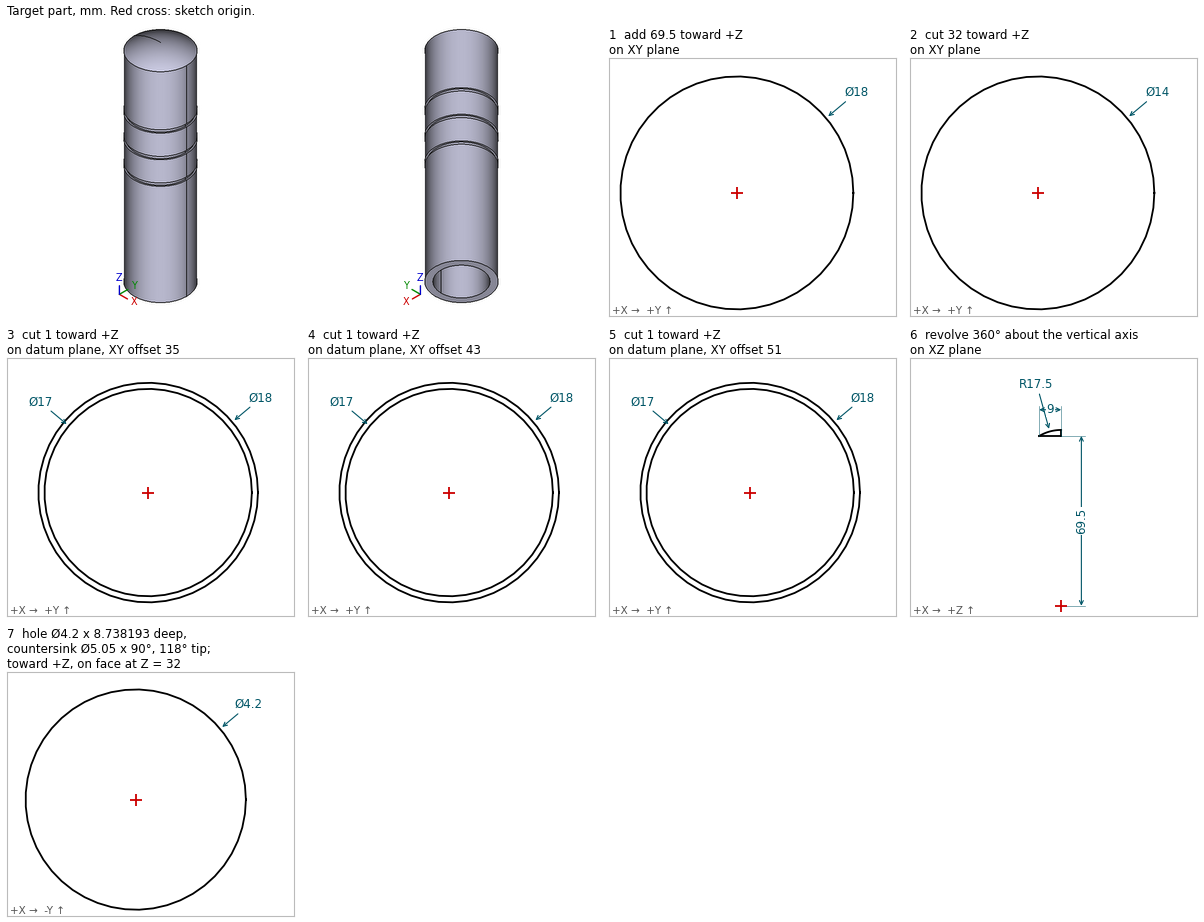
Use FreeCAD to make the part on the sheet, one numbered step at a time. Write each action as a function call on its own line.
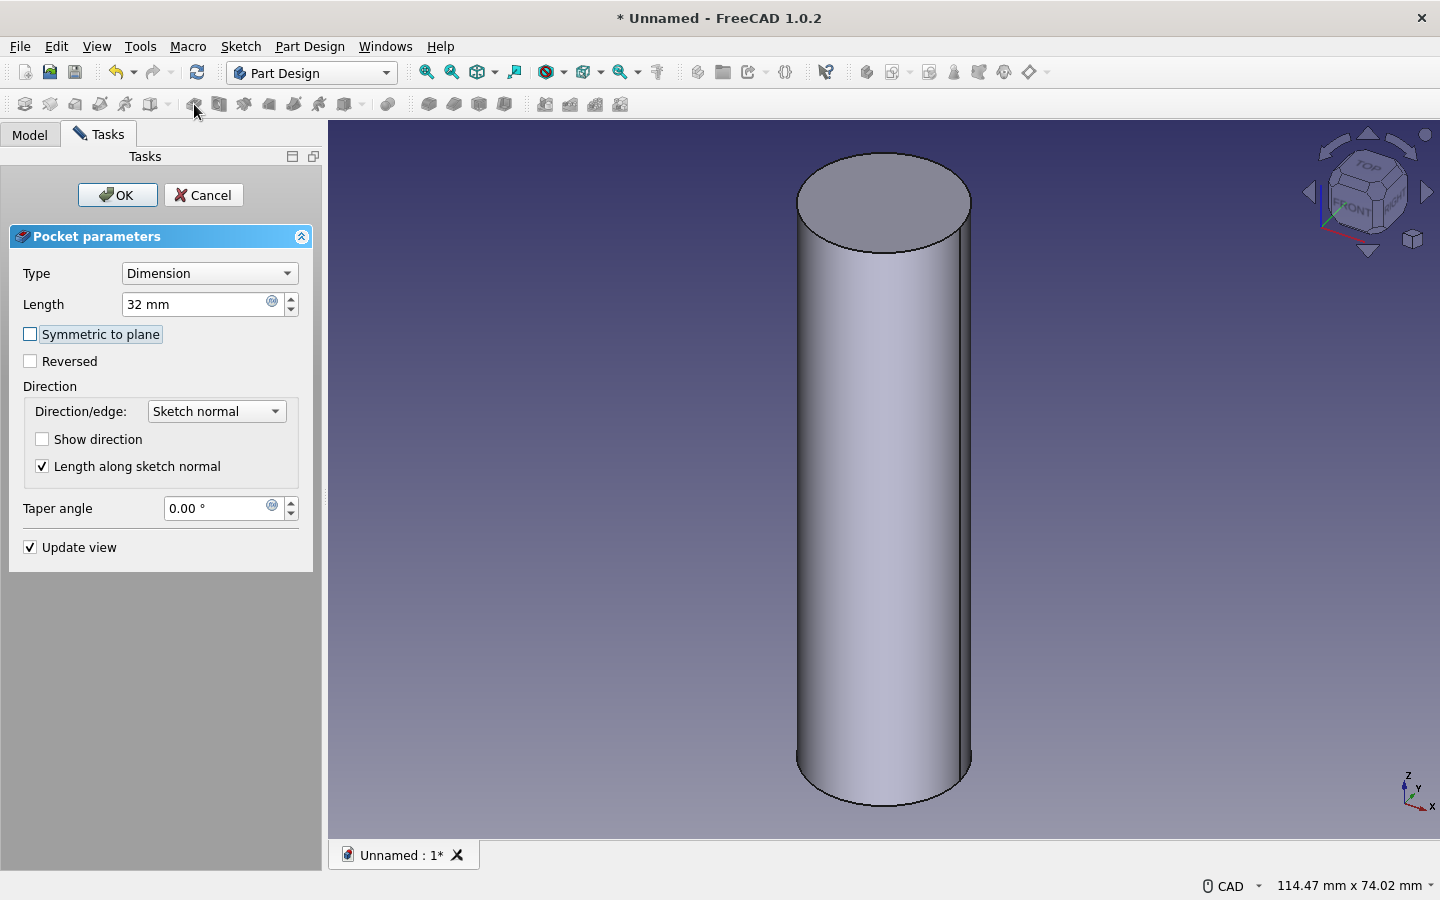
click(31, 361)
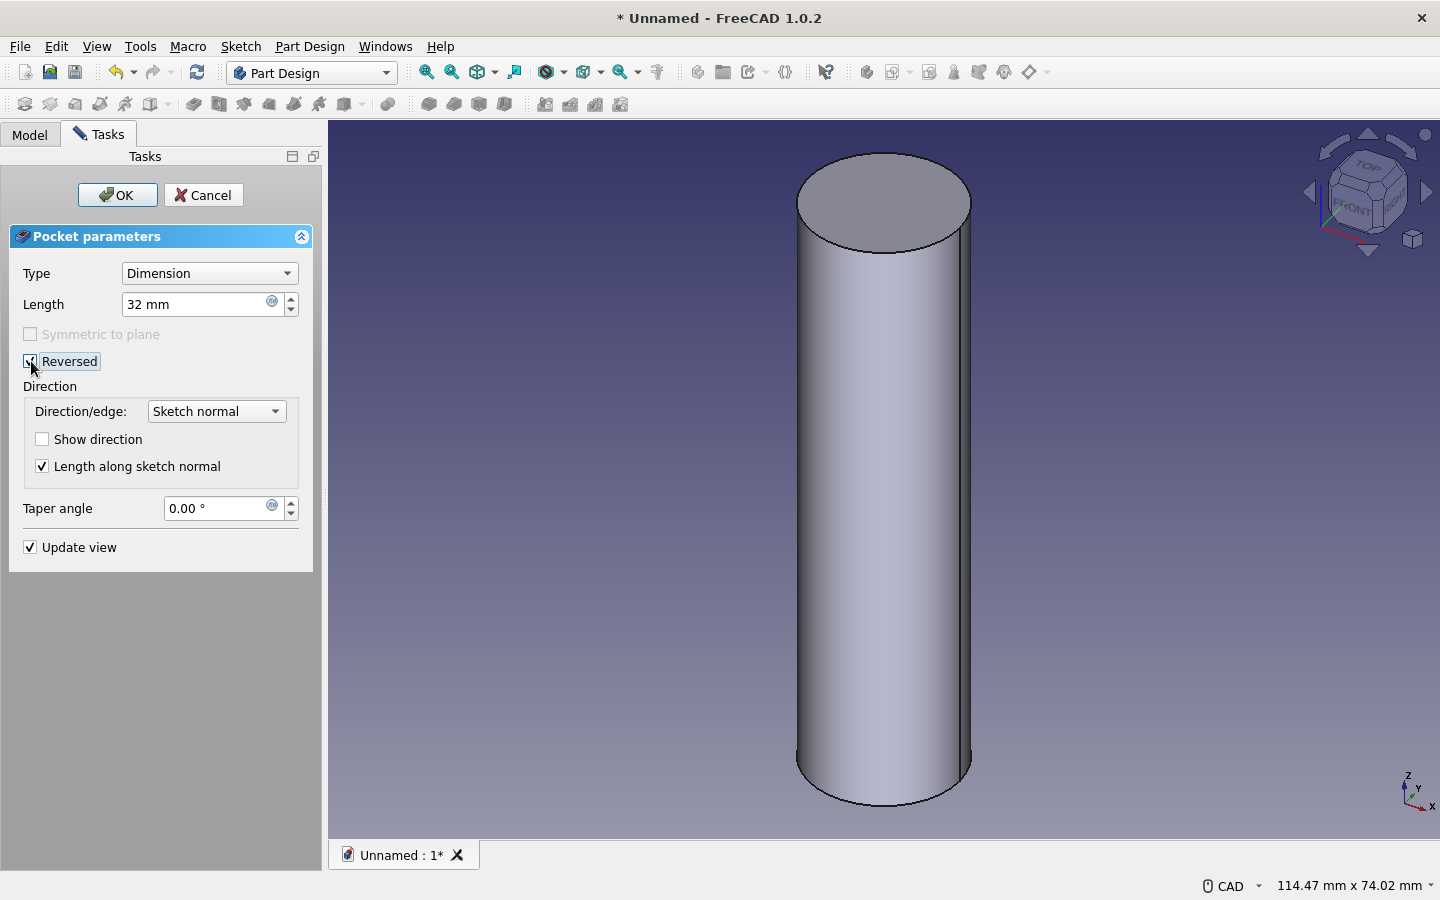
click(118, 195)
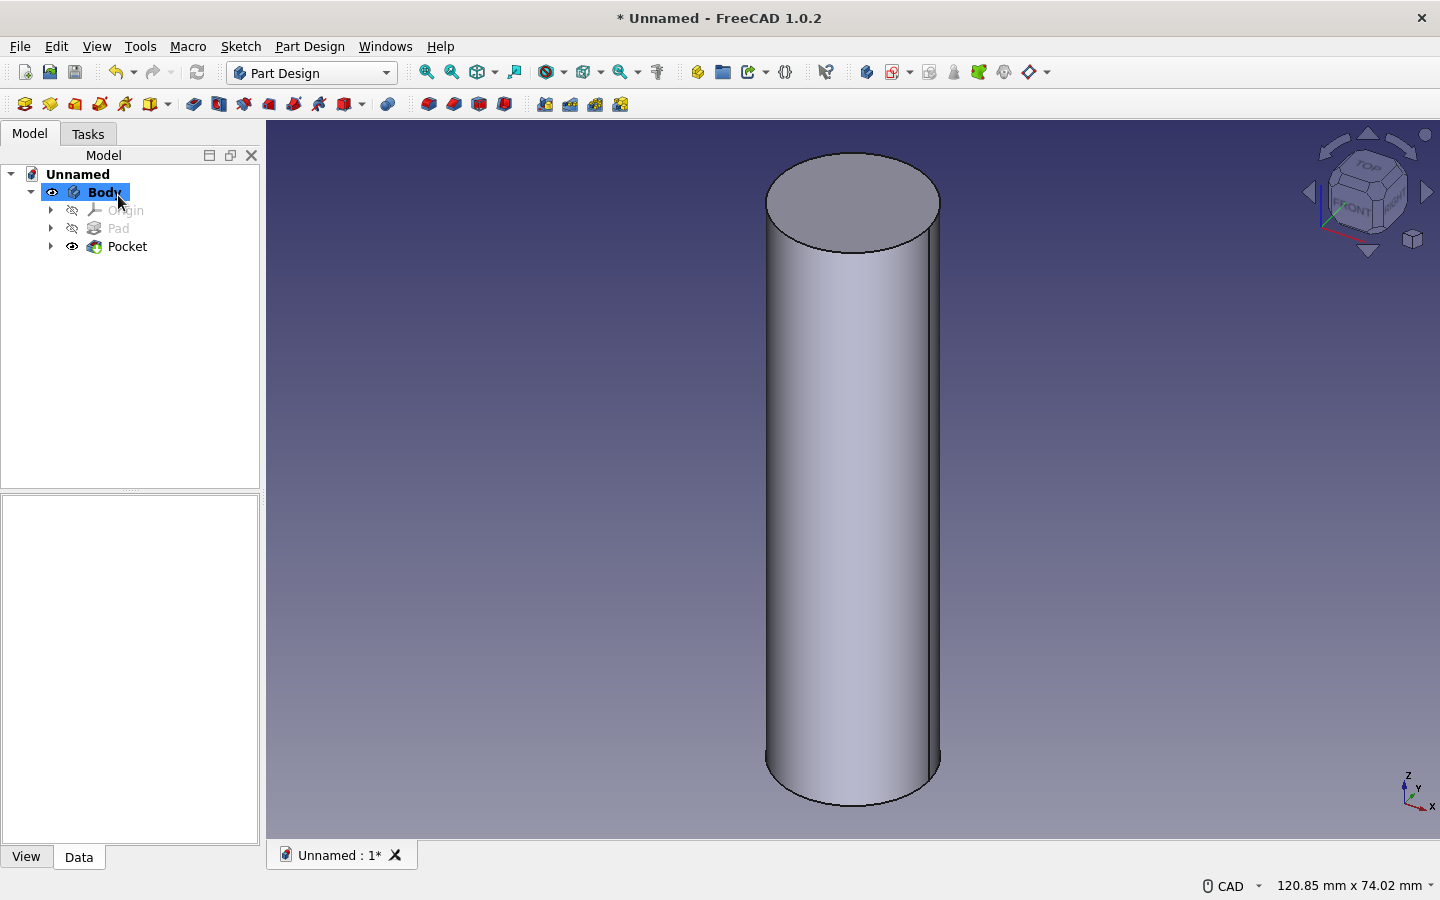
click(51, 210)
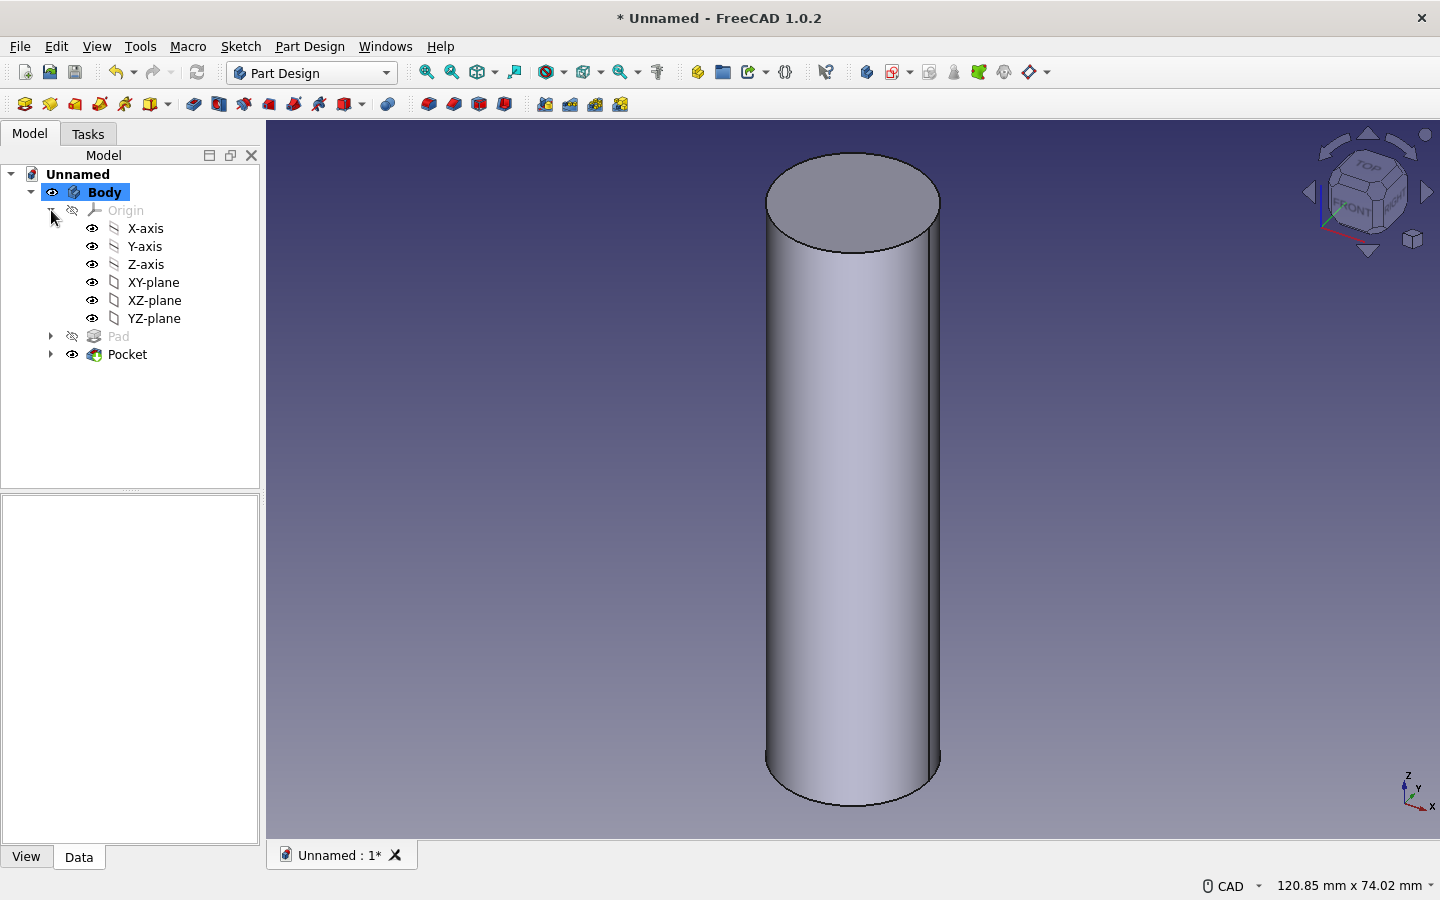
click(137, 282)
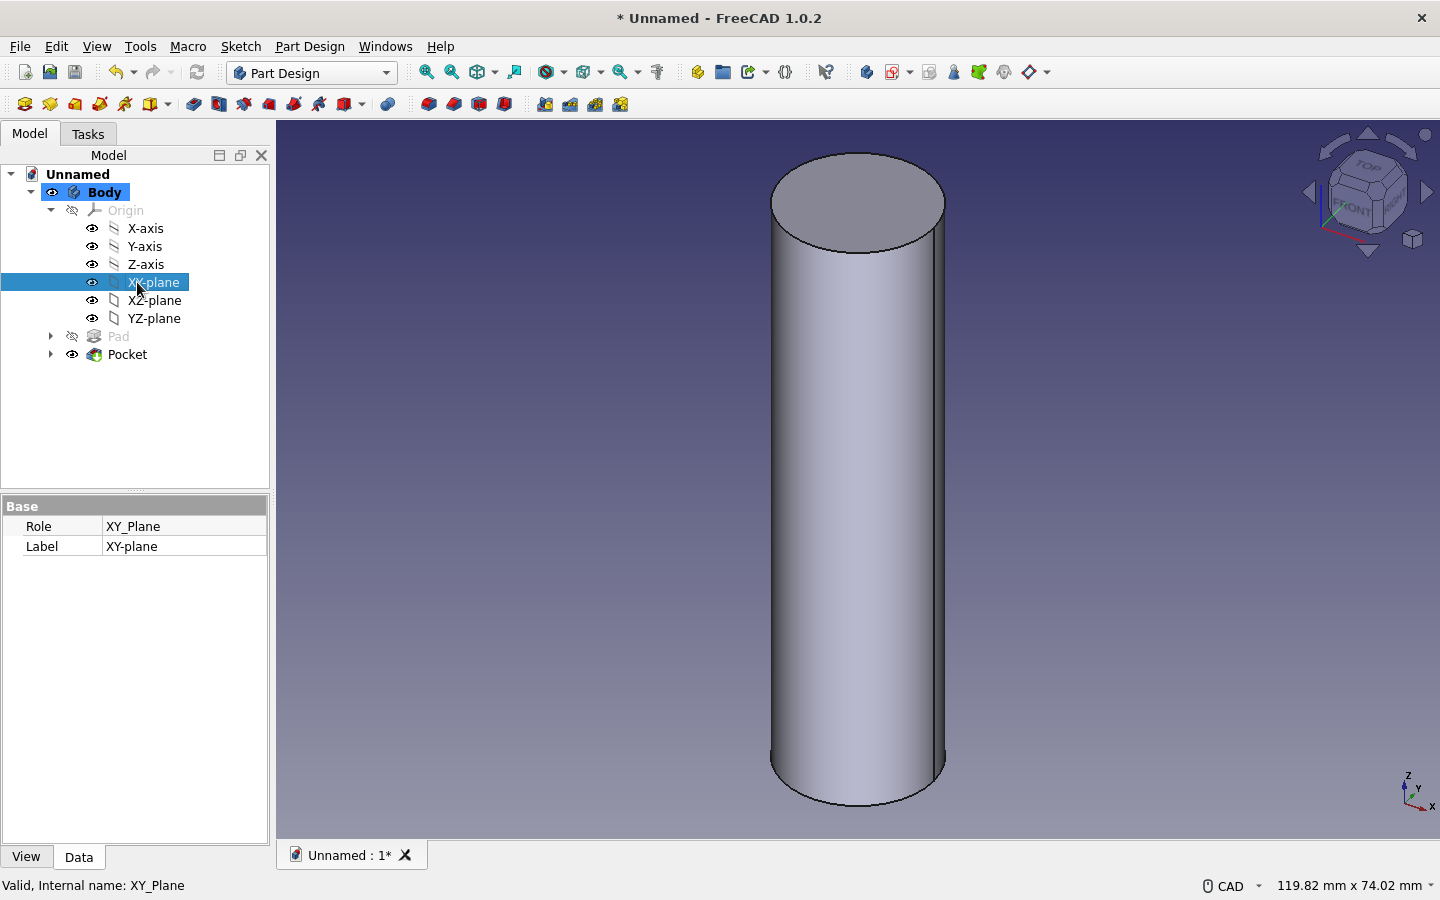
click(1028, 72)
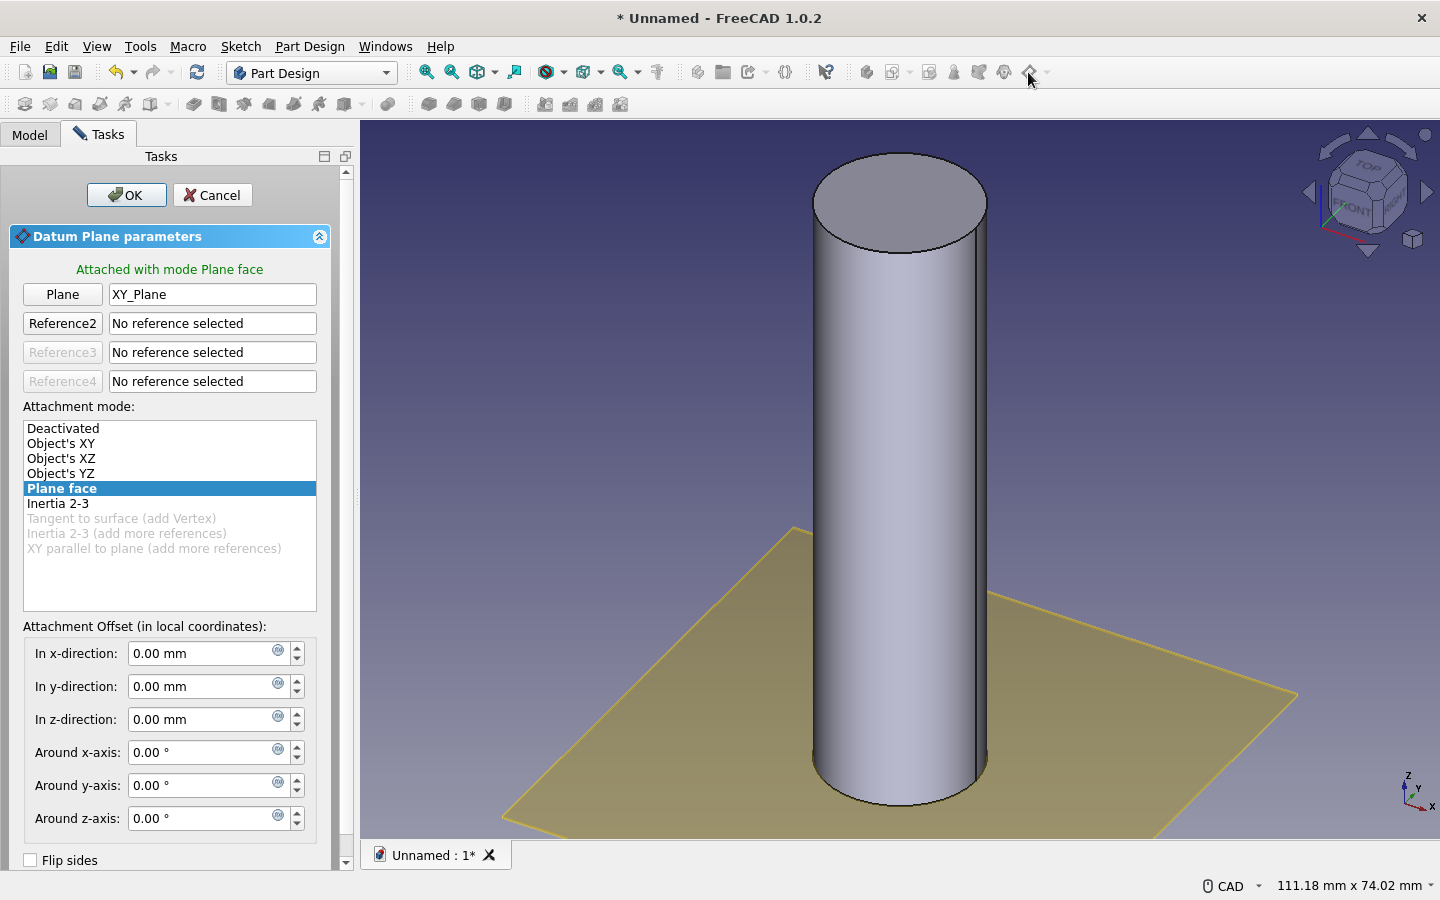
triple_click(210, 720)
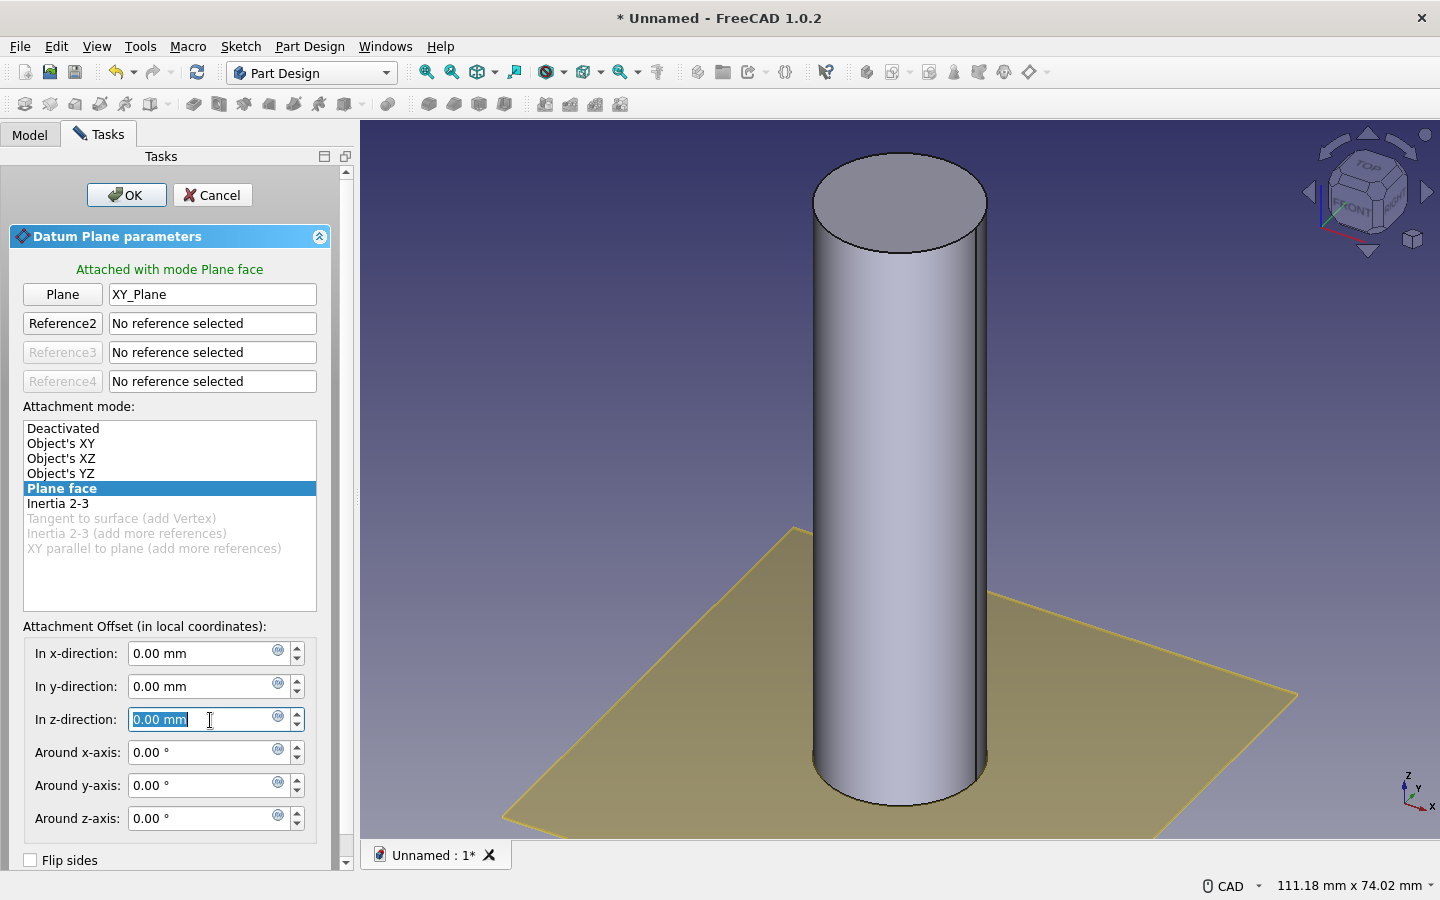
text(35)
key(Tab)